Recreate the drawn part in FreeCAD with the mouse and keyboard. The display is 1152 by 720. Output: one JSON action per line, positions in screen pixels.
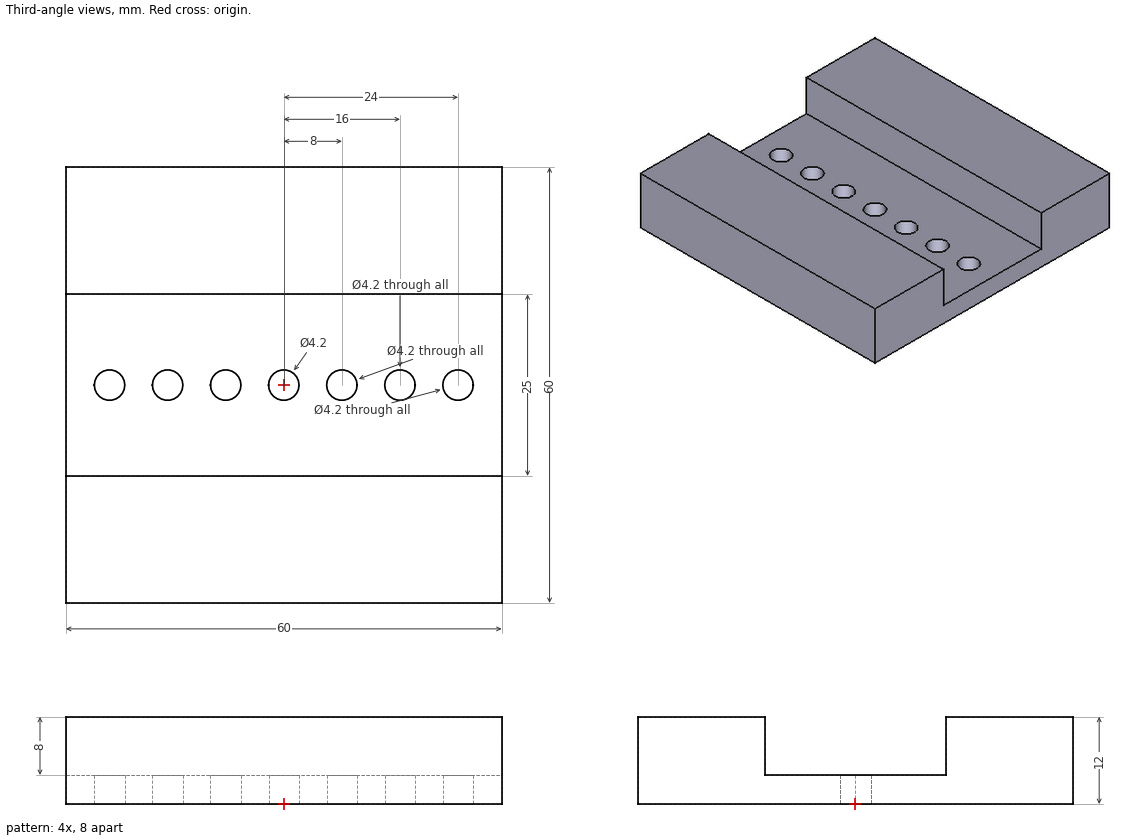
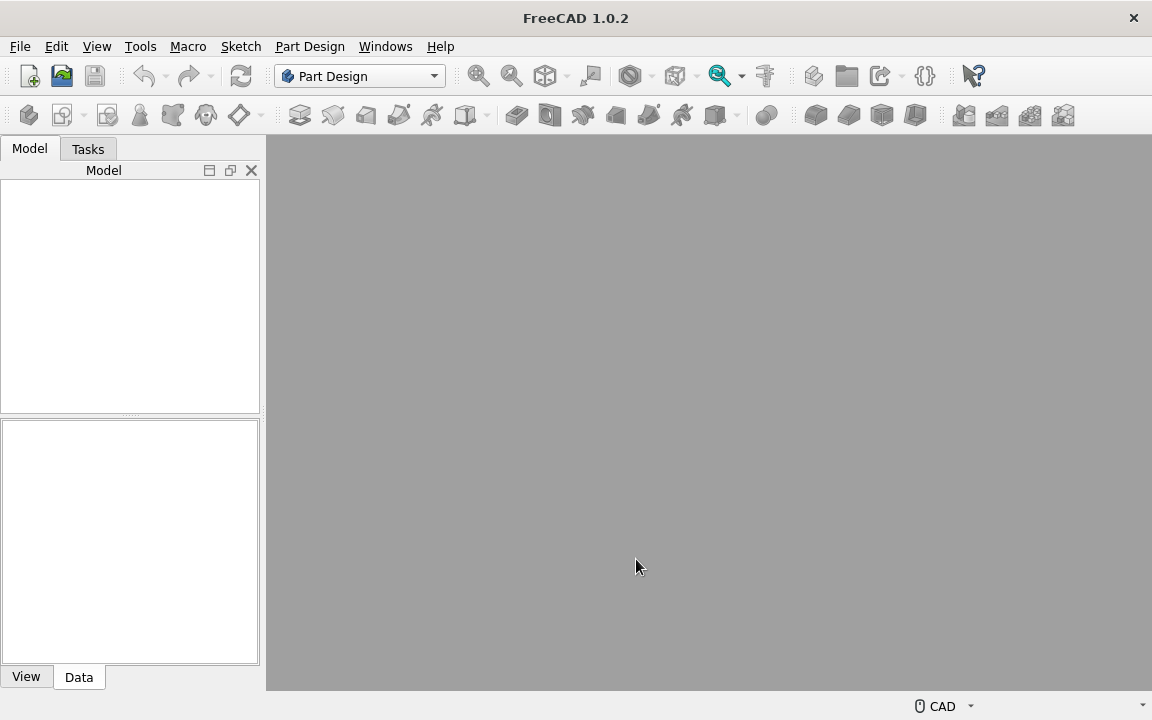
{"action": "left_click", "coordinate": [29, 76]}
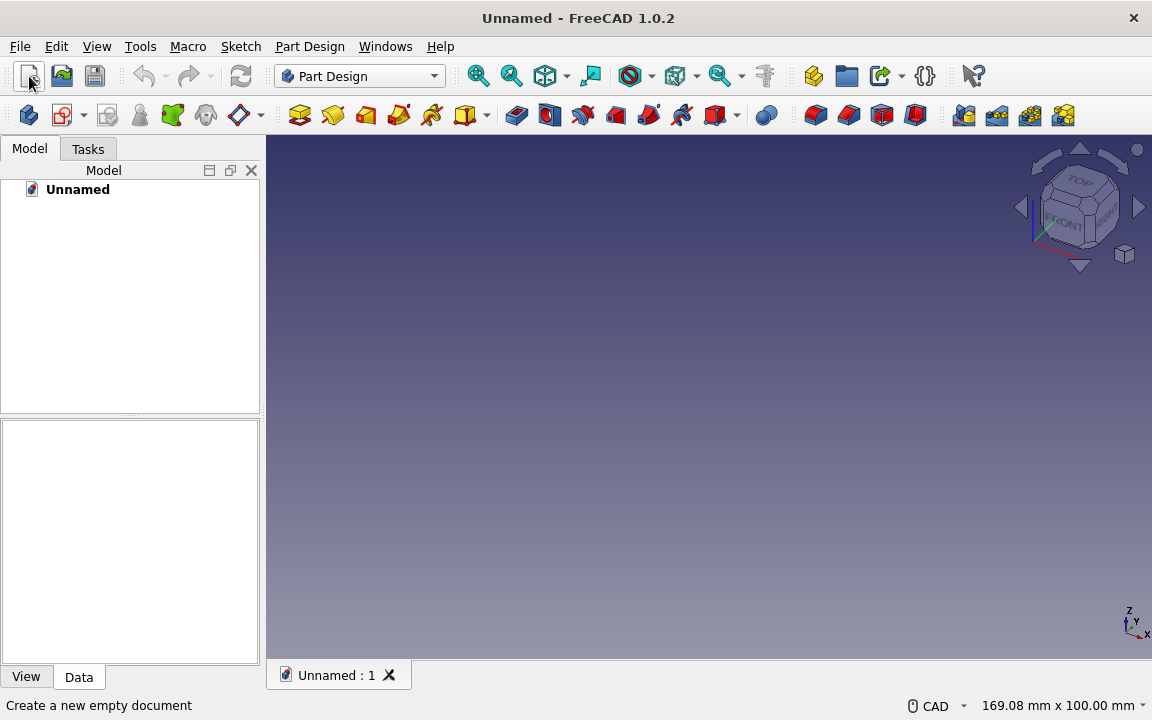
{"action": "left_click", "coordinate": [62, 116]}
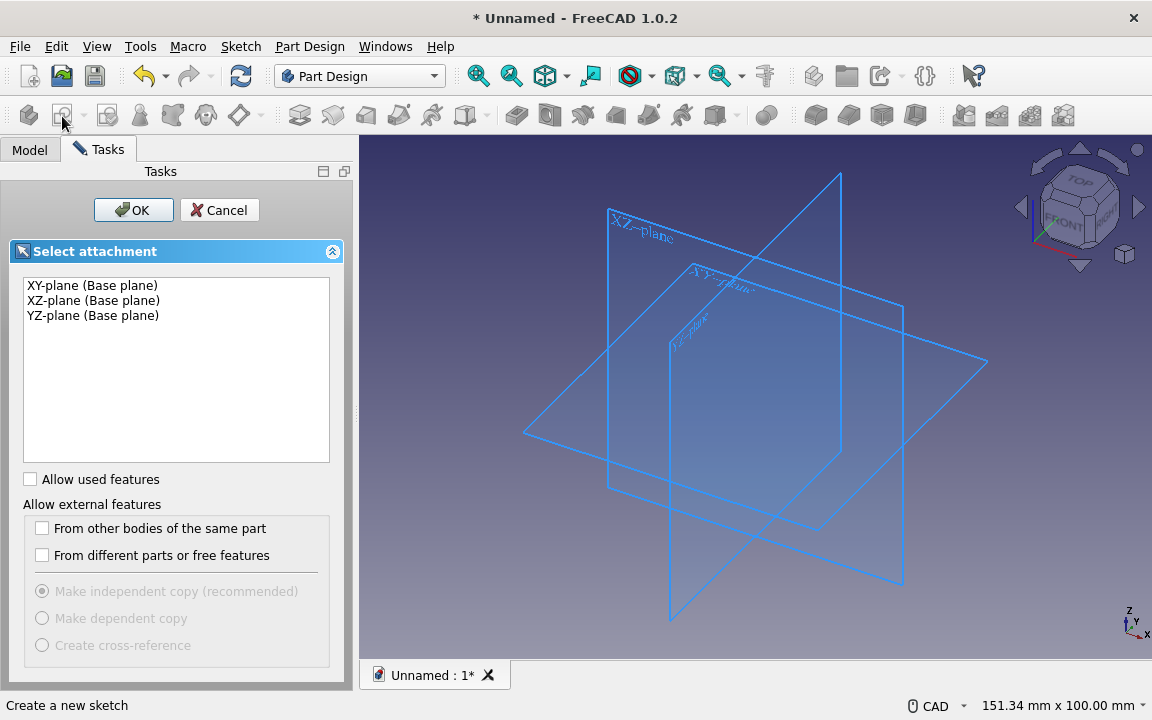
{"action": "left_click", "coordinate": [84, 286]}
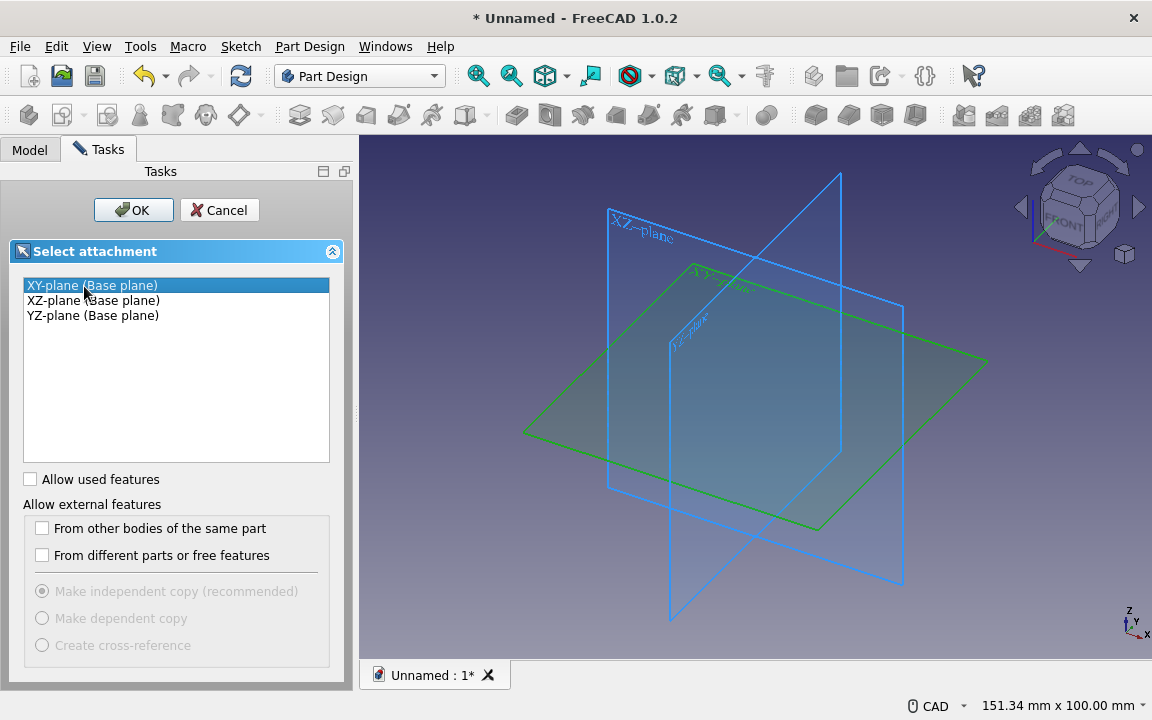
{"action": "left_click", "coordinate": [134, 210]}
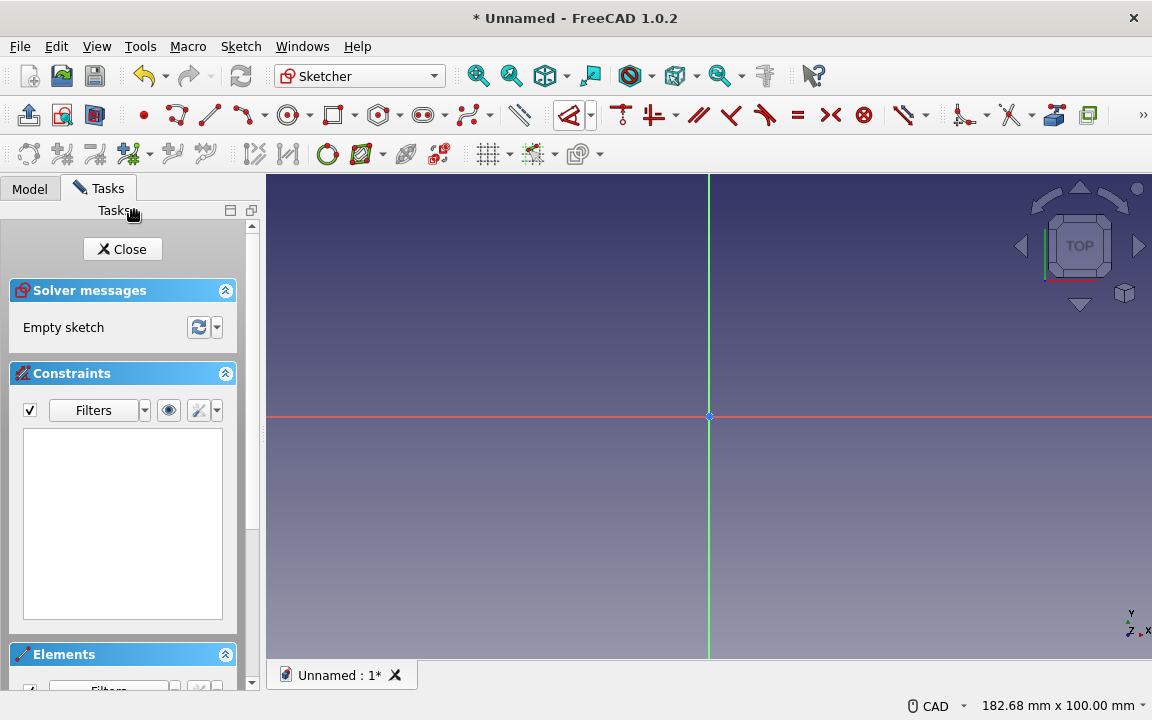
{"action": "key", "text": "g v"}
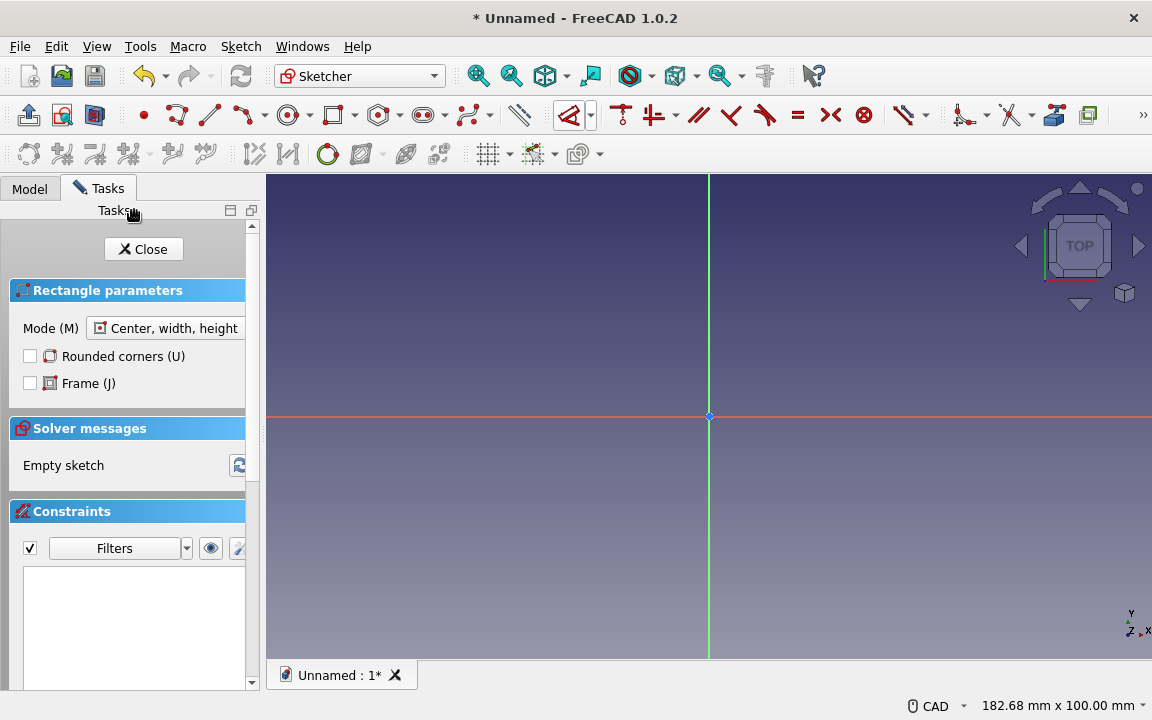
{"action": "left_click", "coordinate": [709, 416]}
{"action": "mouse_move", "coordinate": [854, 271]}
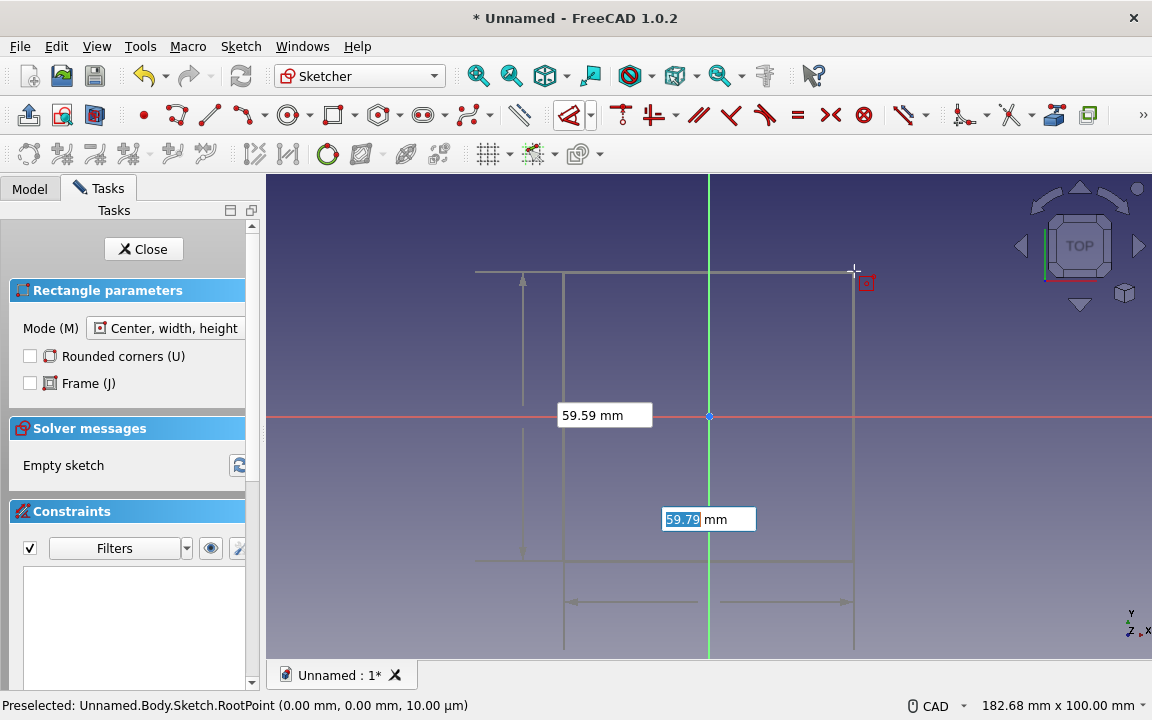
{"action": "type", "text": "60"}
{"action": "key", "text": "Tab"}
{"action": "type", "text": "60"}
{"action": "key", "text": "Return"}
{"action": "key", "text": "Escape"}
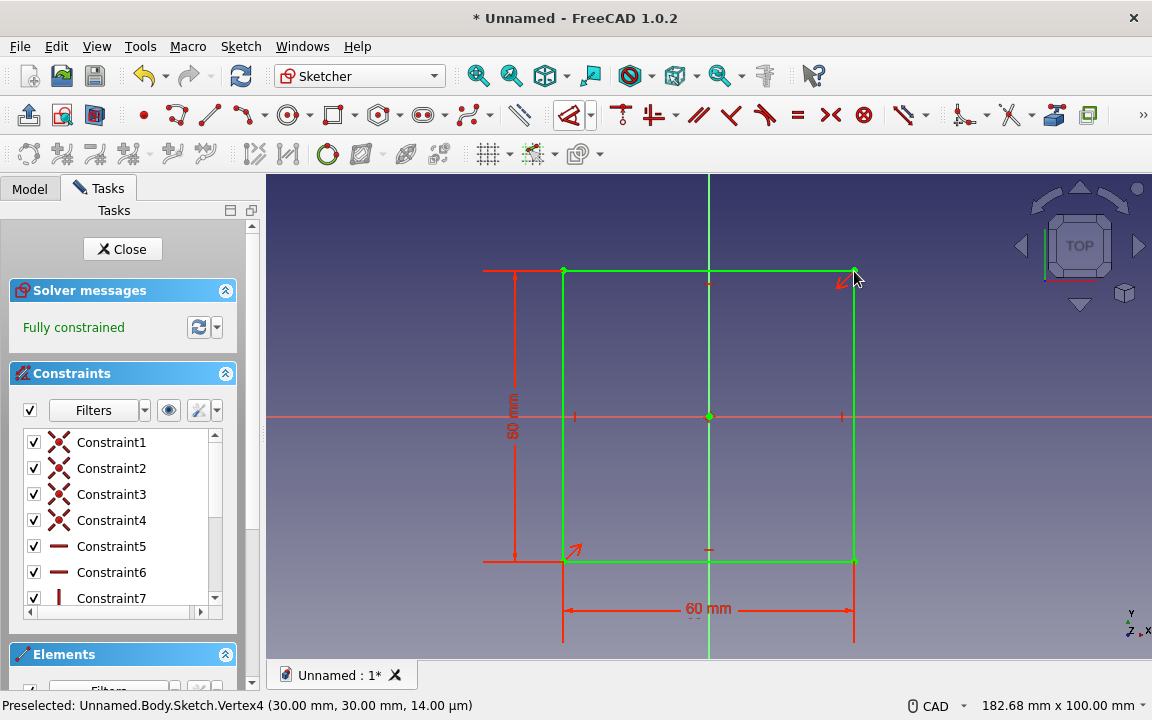
{"action": "left_click", "coordinate": [123, 249]}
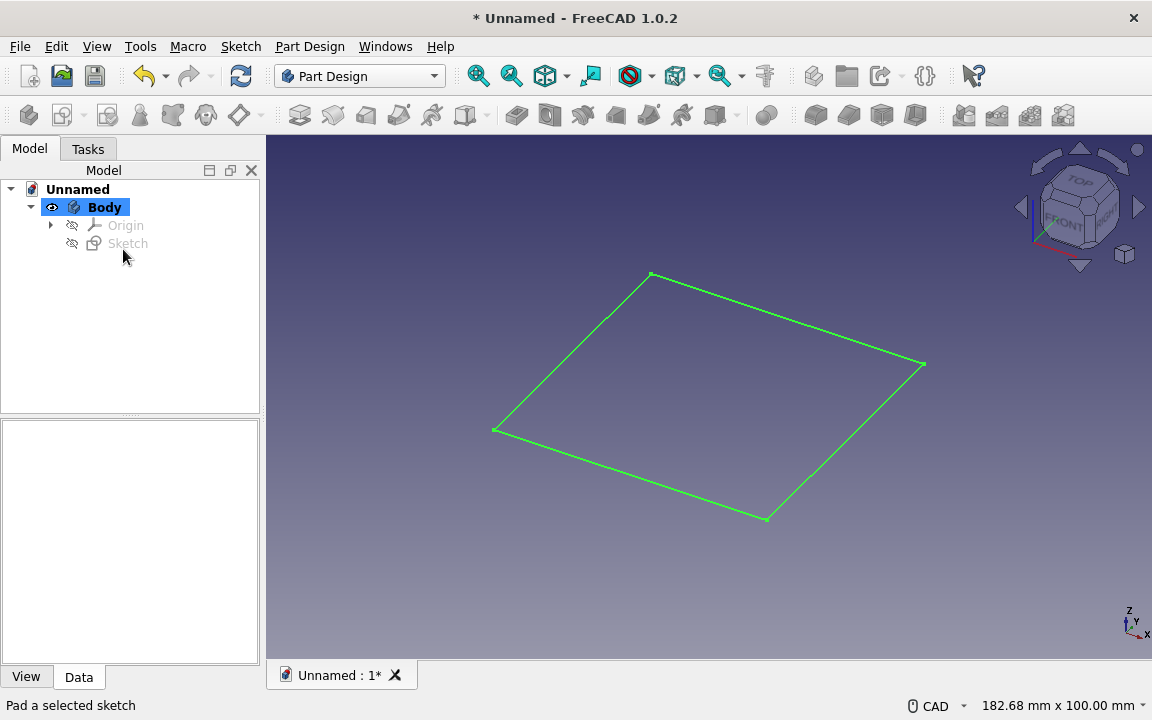
{"action": "left_click", "coordinate": [300, 116]}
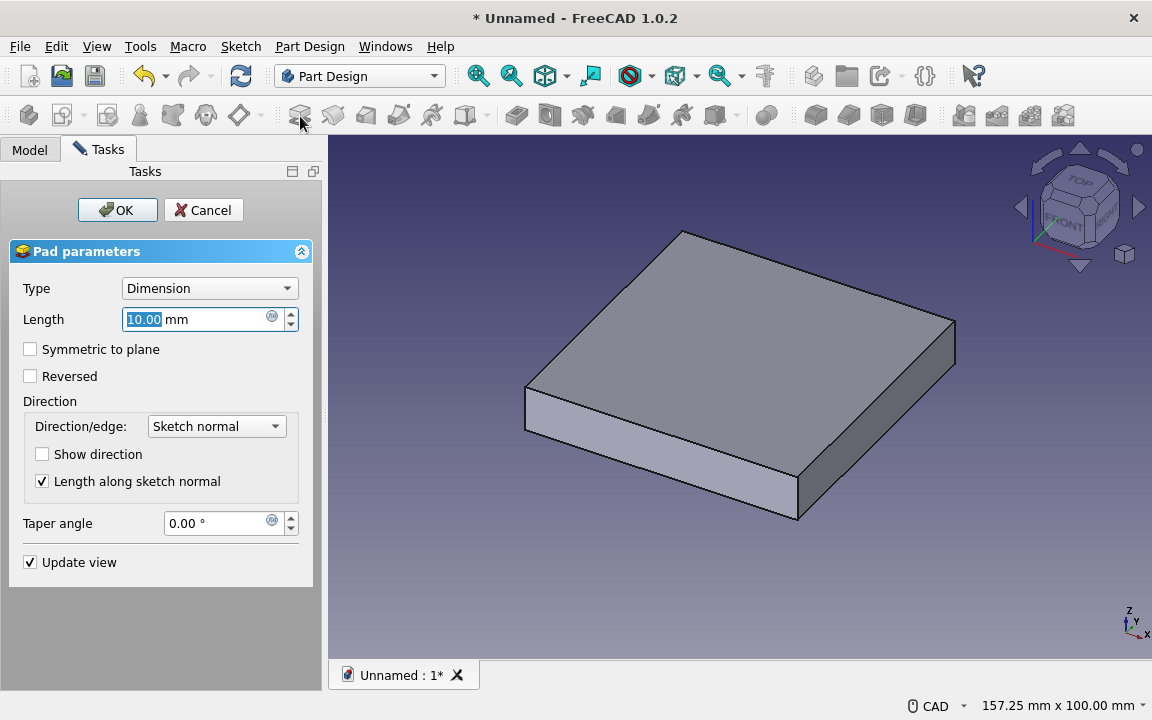
{"action": "type", "text": "12"}
{"action": "key", "text": "Tab"}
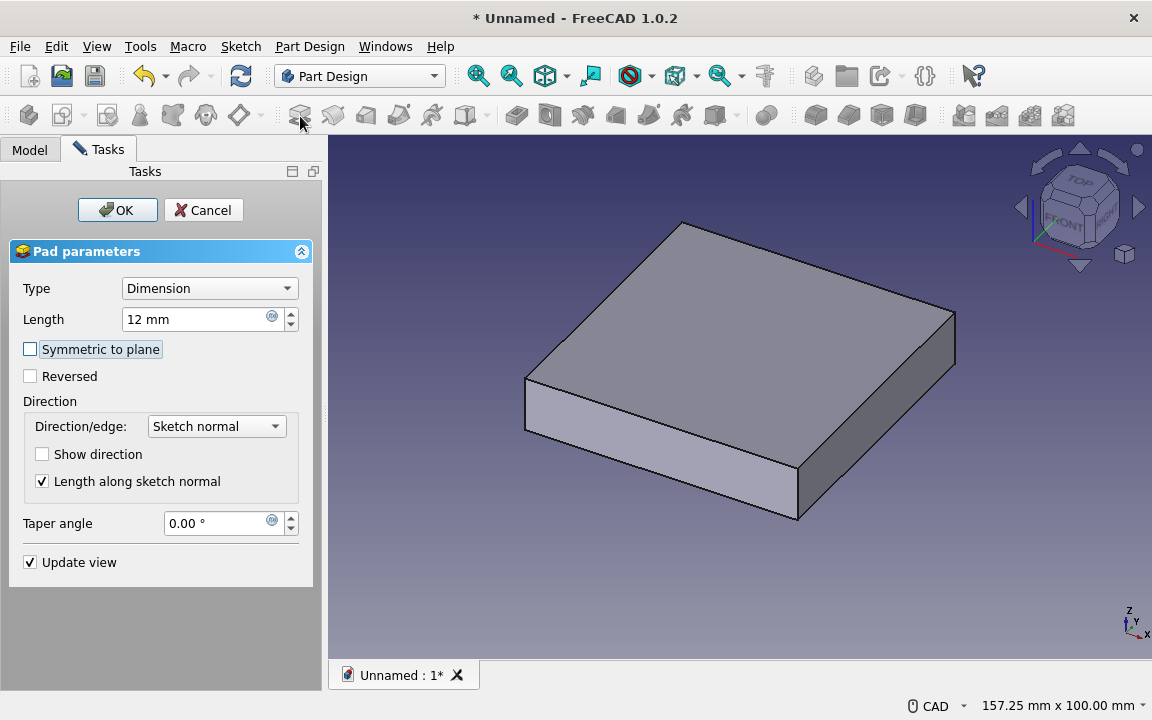
{"action": "left_click", "coordinate": [118, 210]}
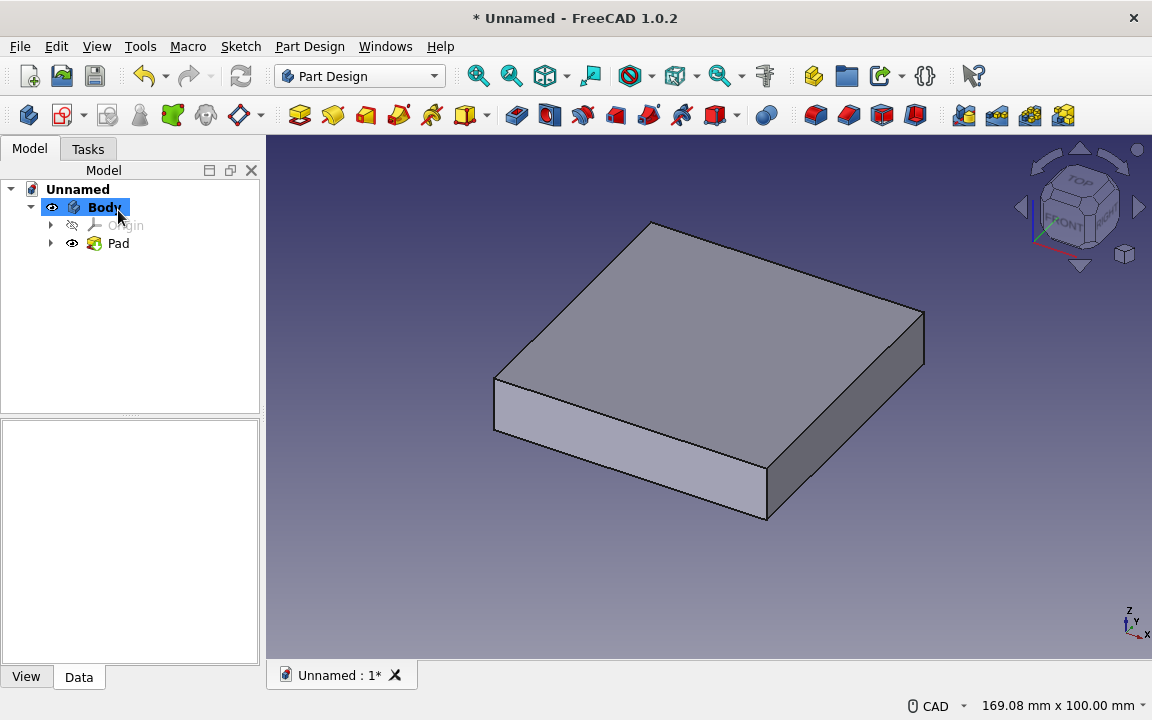
{"action": "left_click", "coordinate": [709, 344]}